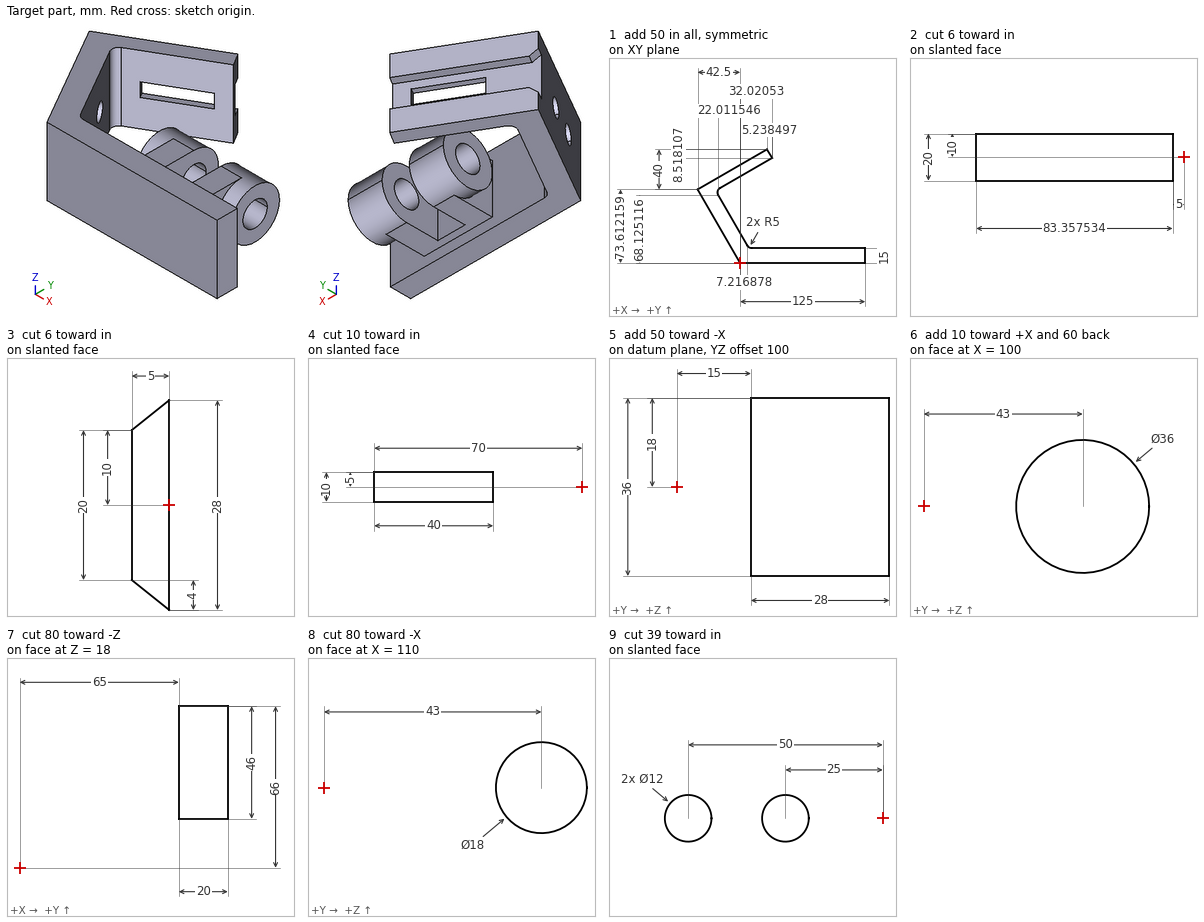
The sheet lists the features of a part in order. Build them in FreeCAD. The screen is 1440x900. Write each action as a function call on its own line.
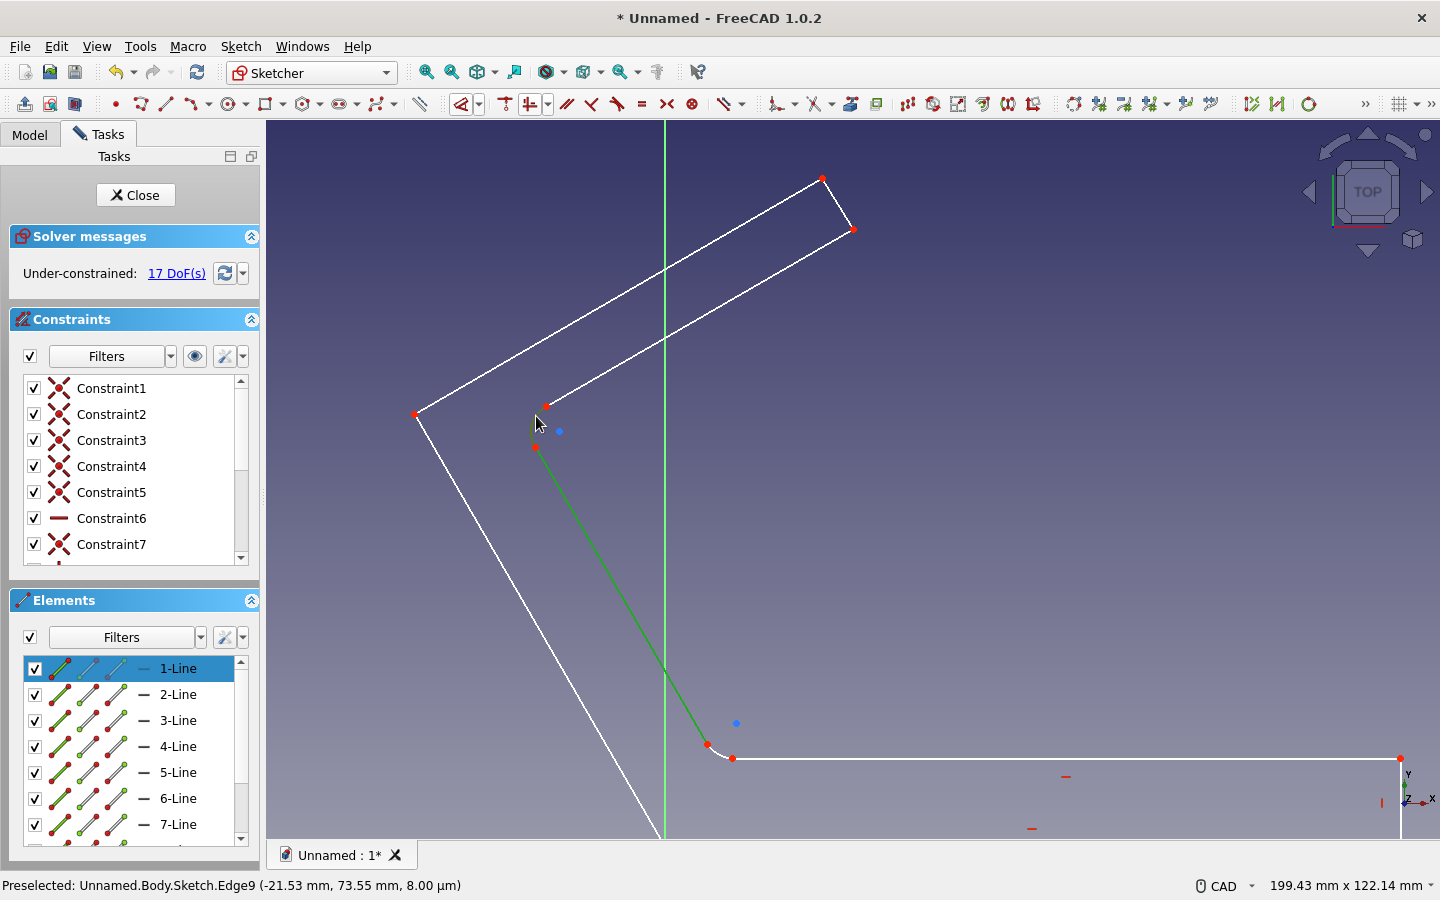
click(617, 104)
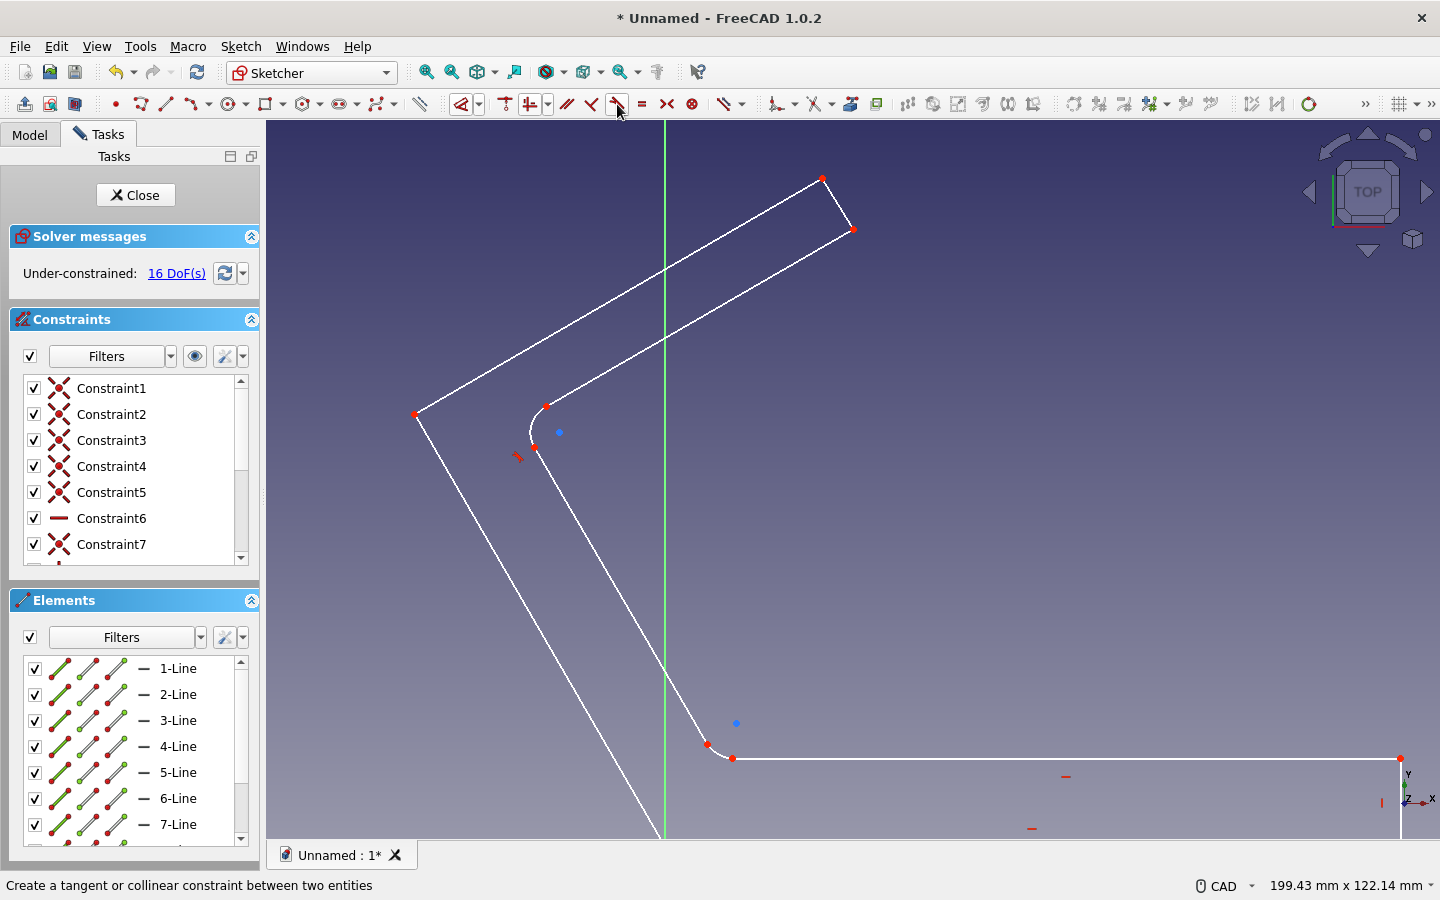
scroll(655, 655, up, 2)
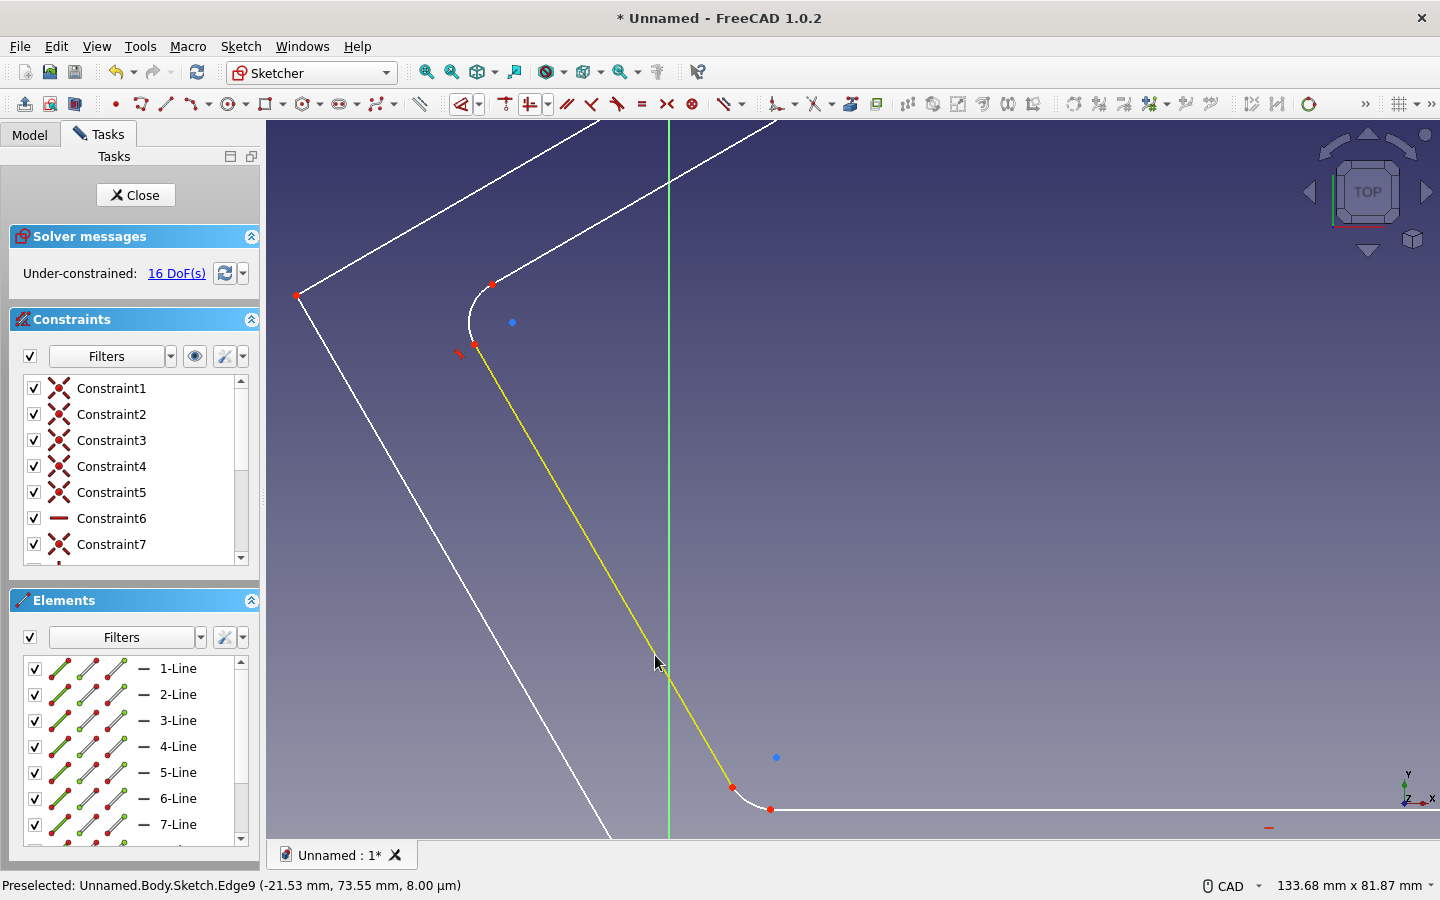
click(655, 655)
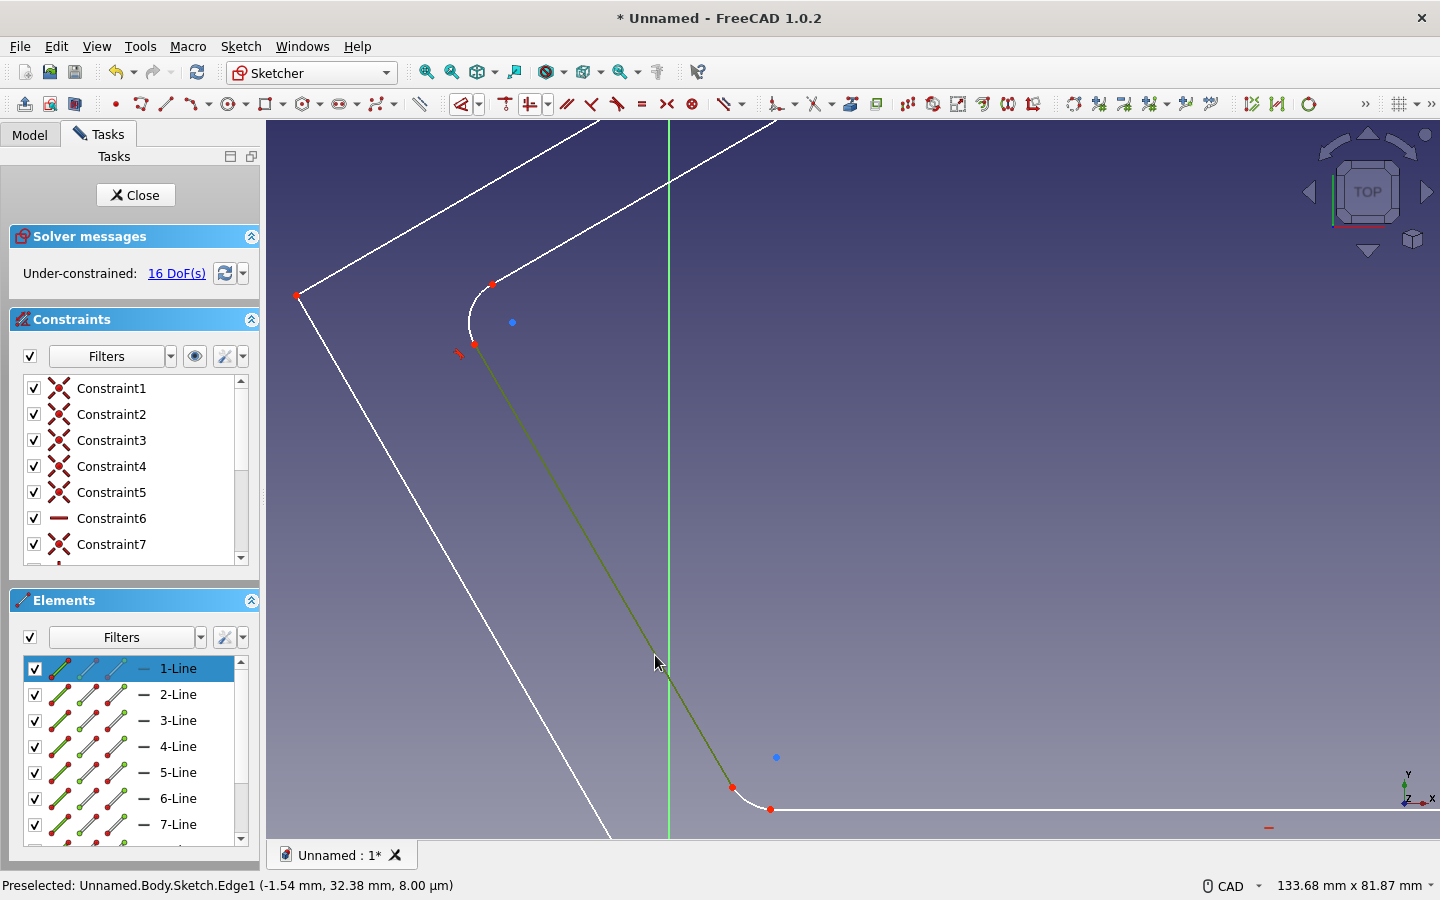
click(742, 797)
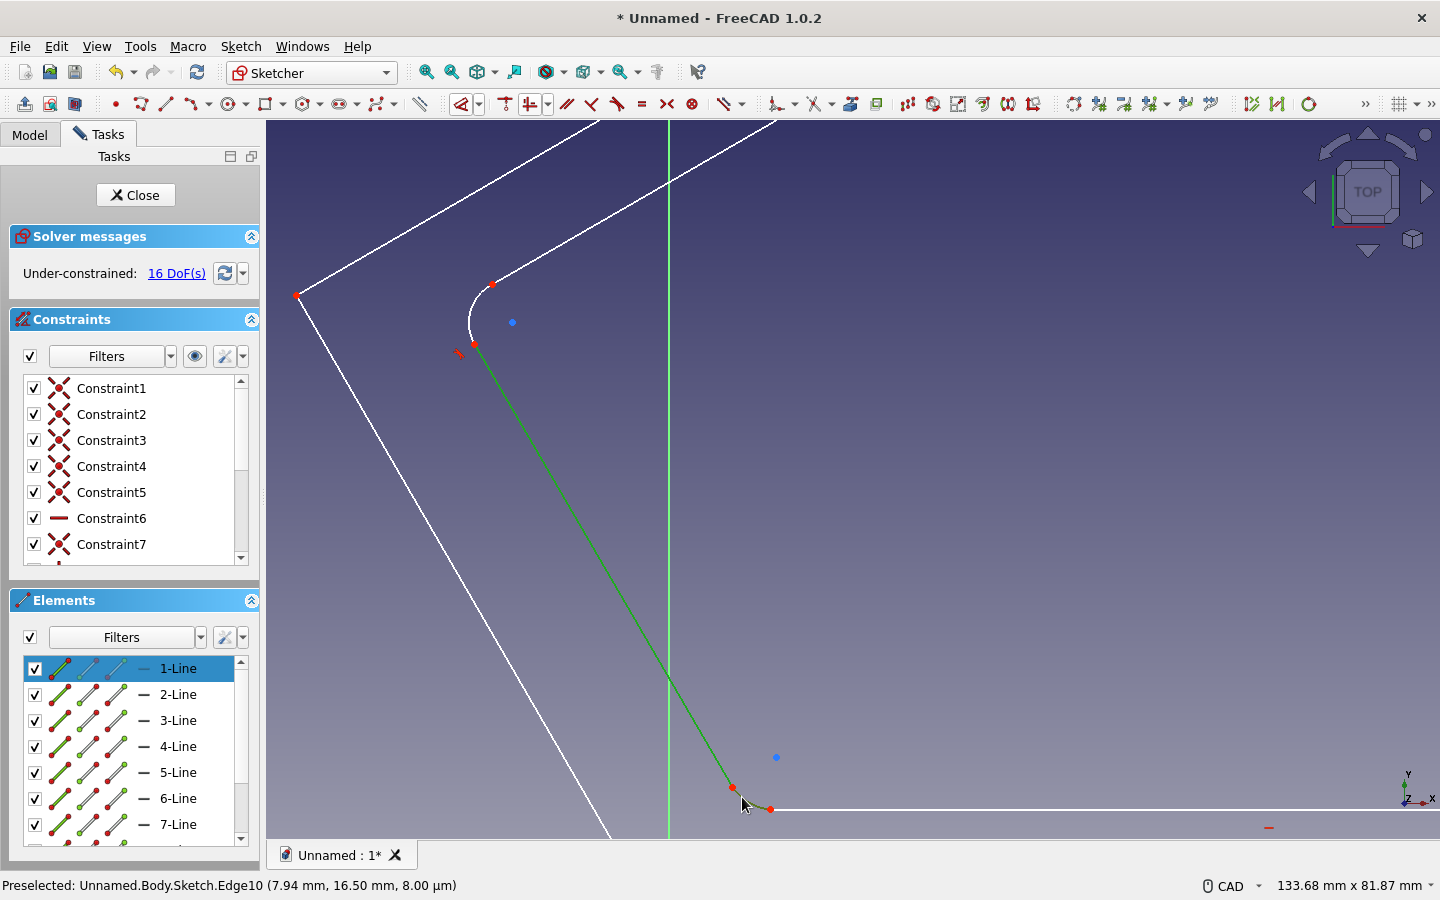
key(t)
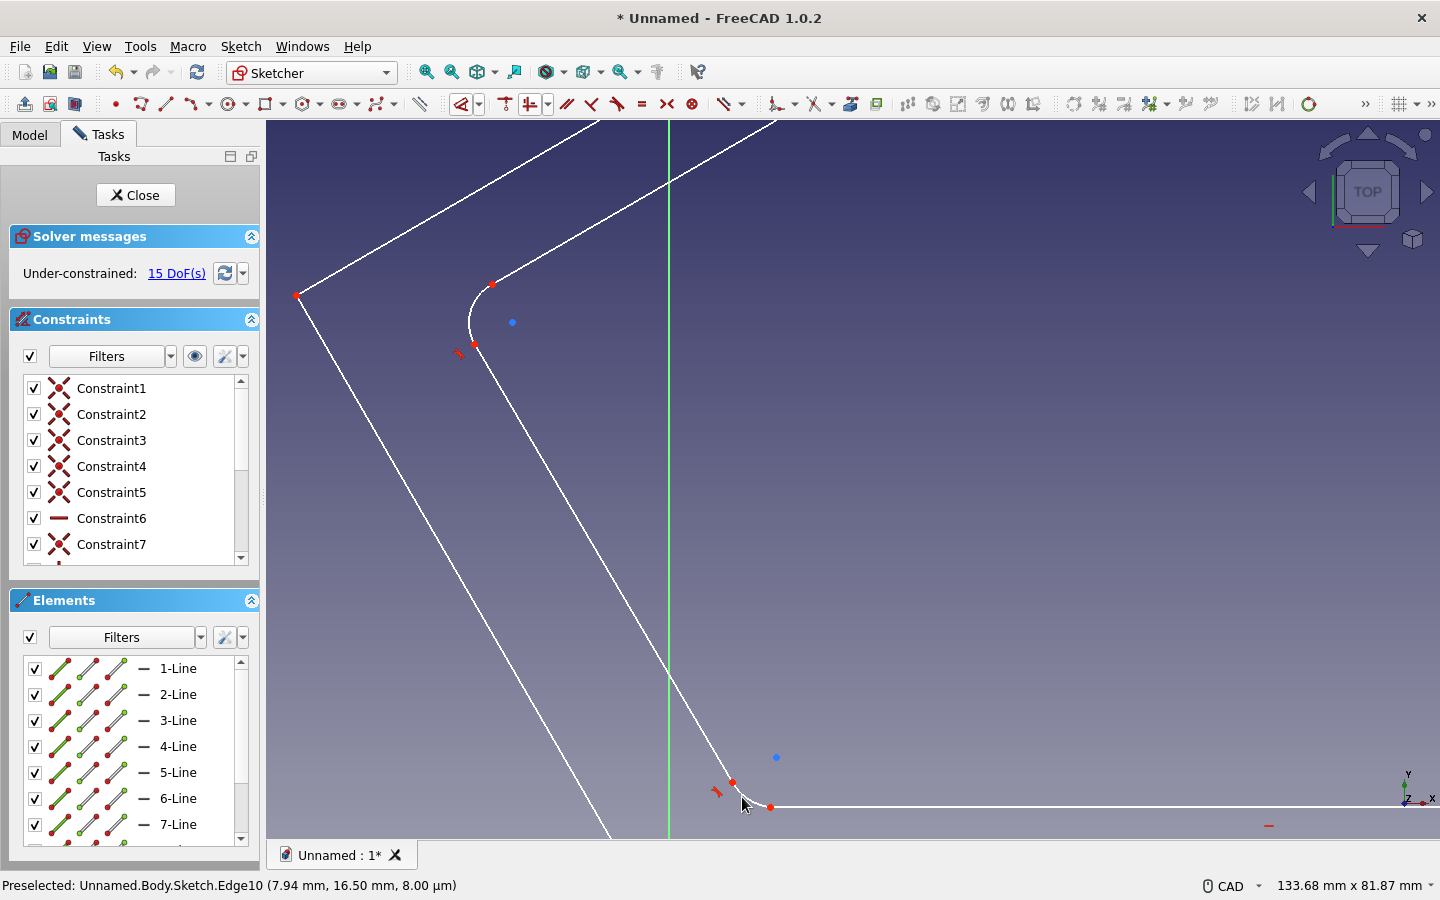
click(630, 205)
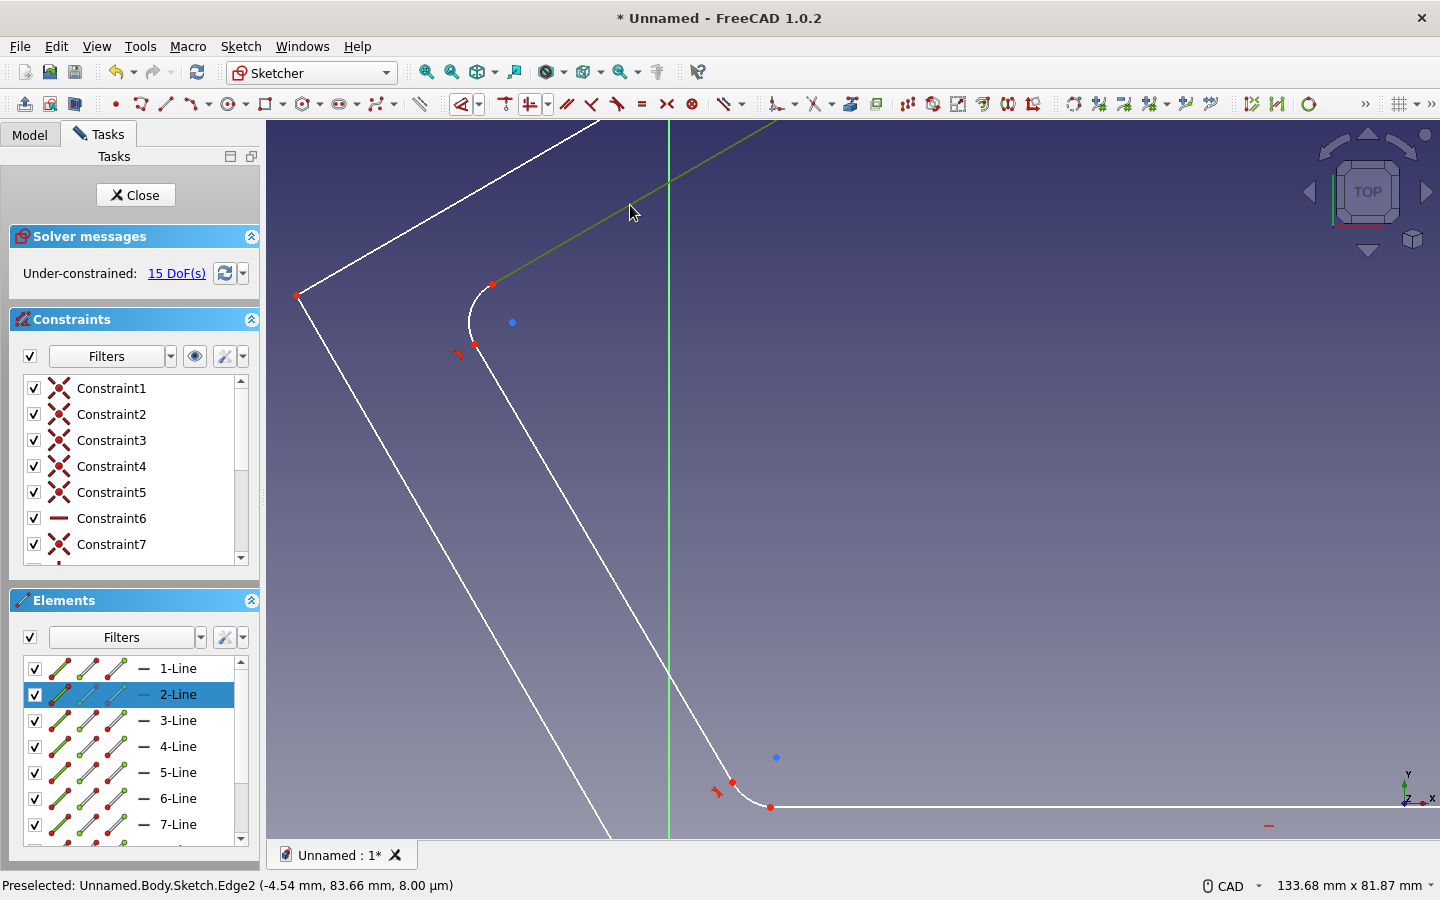
click(477, 298)